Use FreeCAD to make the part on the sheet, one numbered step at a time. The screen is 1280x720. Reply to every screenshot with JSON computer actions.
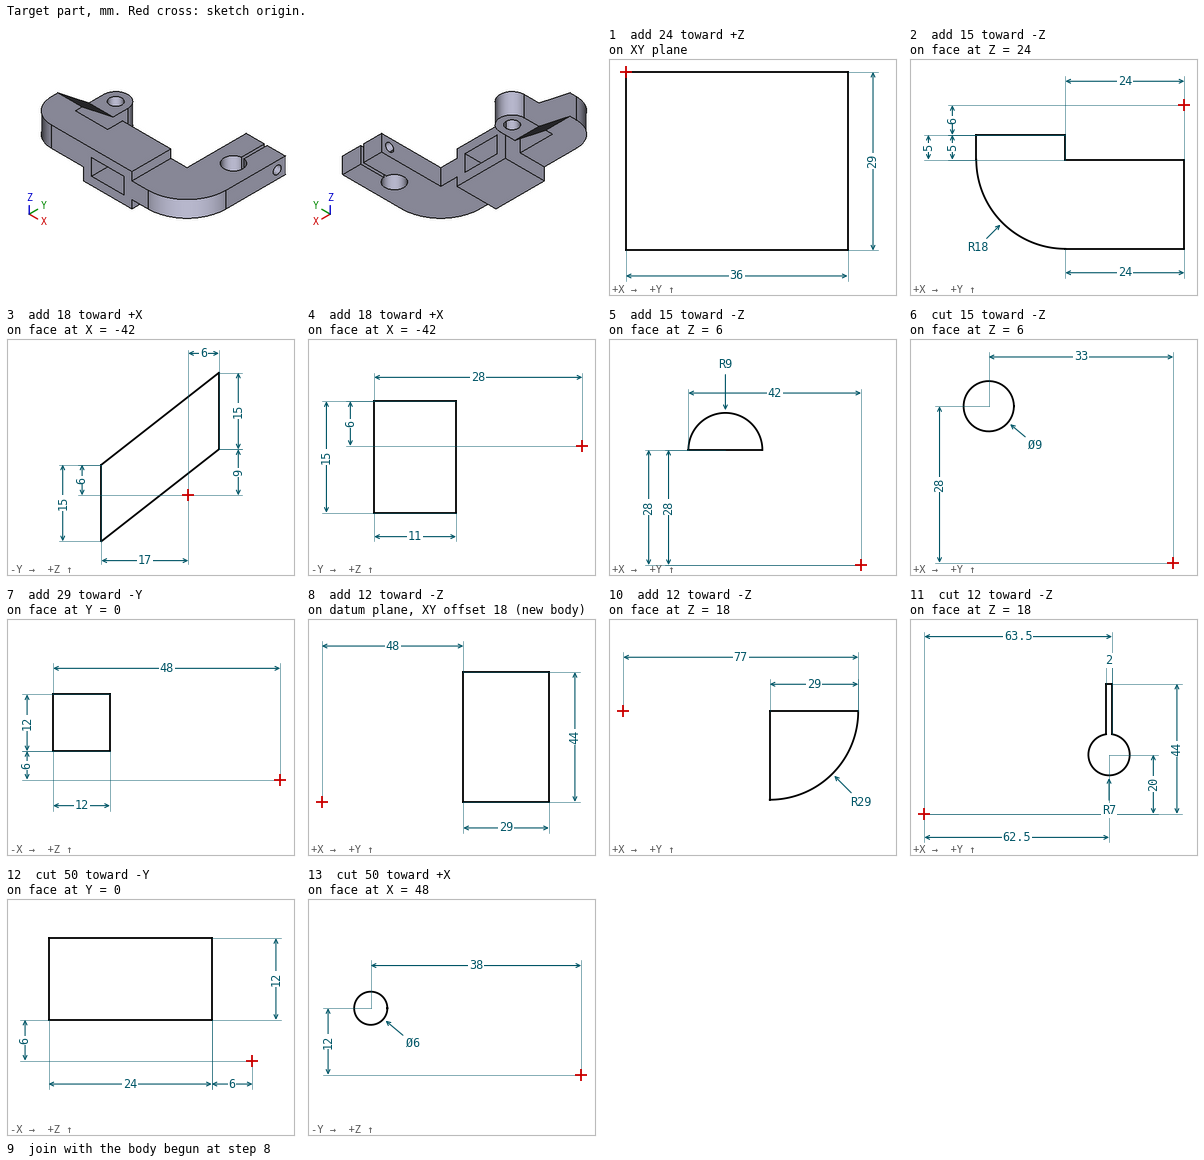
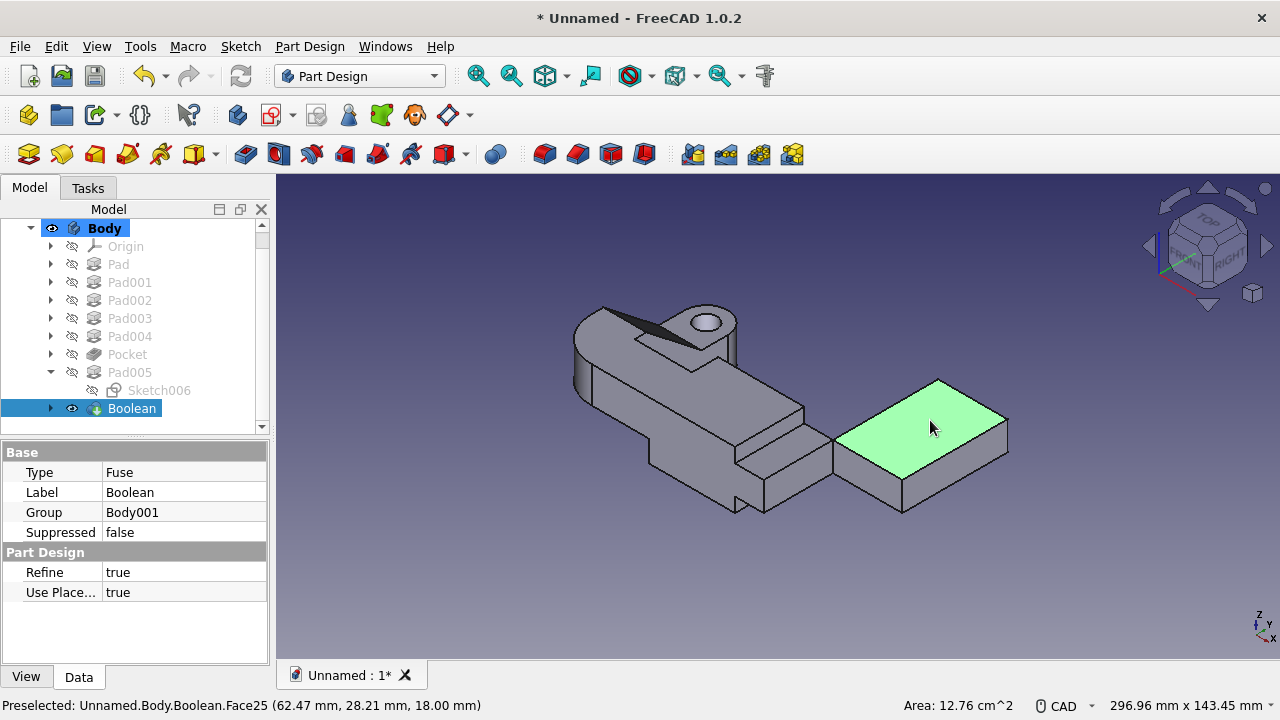
{"action": "left_click", "coordinate": [270, 116]}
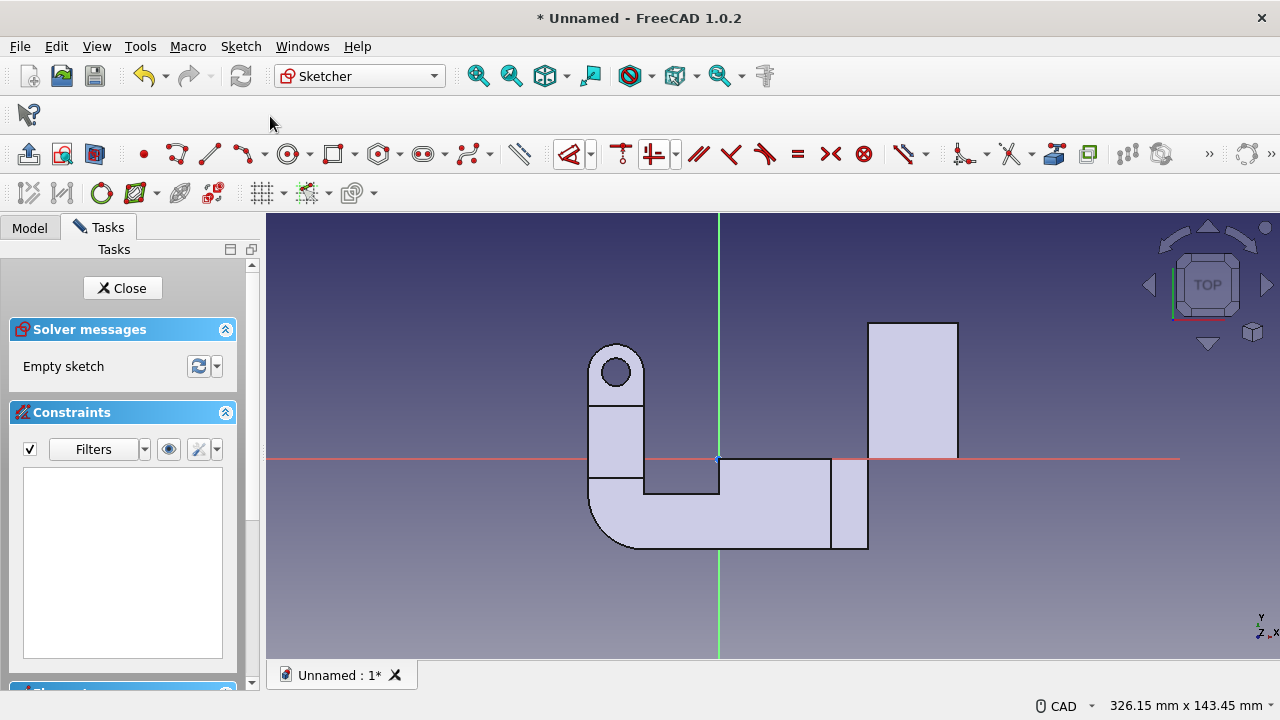
{"action": "scroll", "coordinate": [1003, 534], "scroll_direction": "up", "scroll_amount": 6}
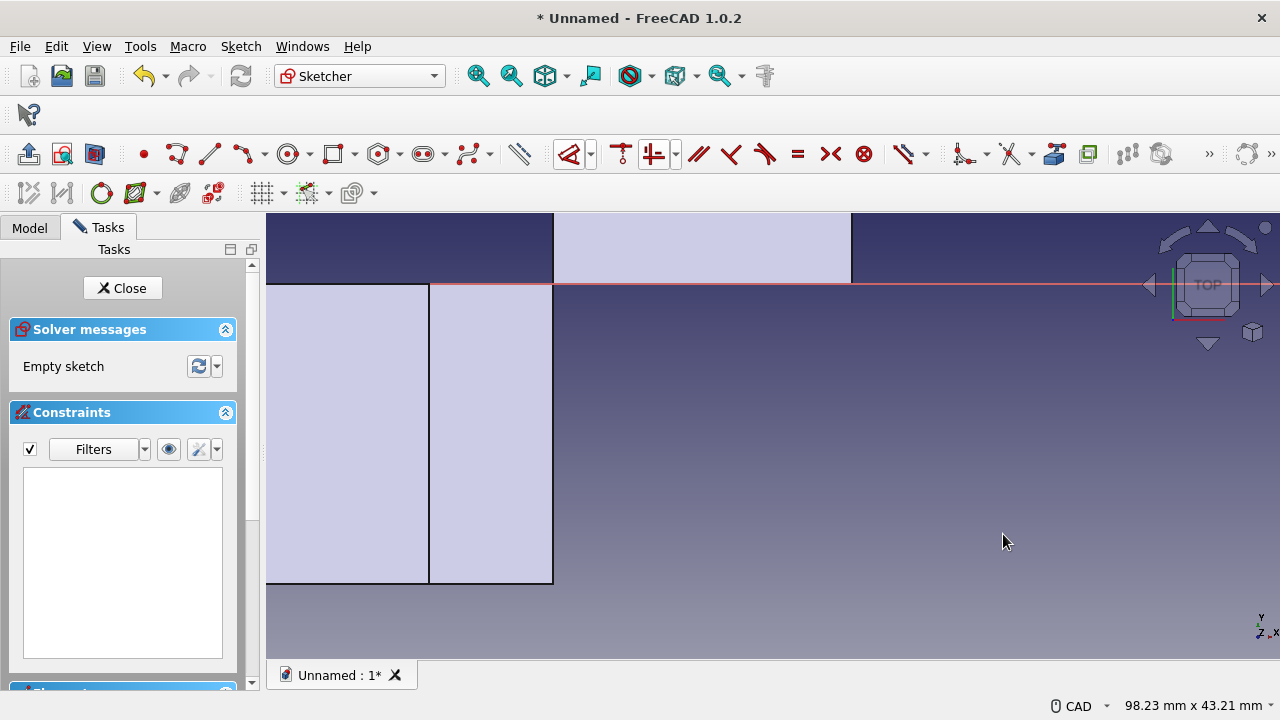
{"action": "left_click", "coordinate": [177, 154]}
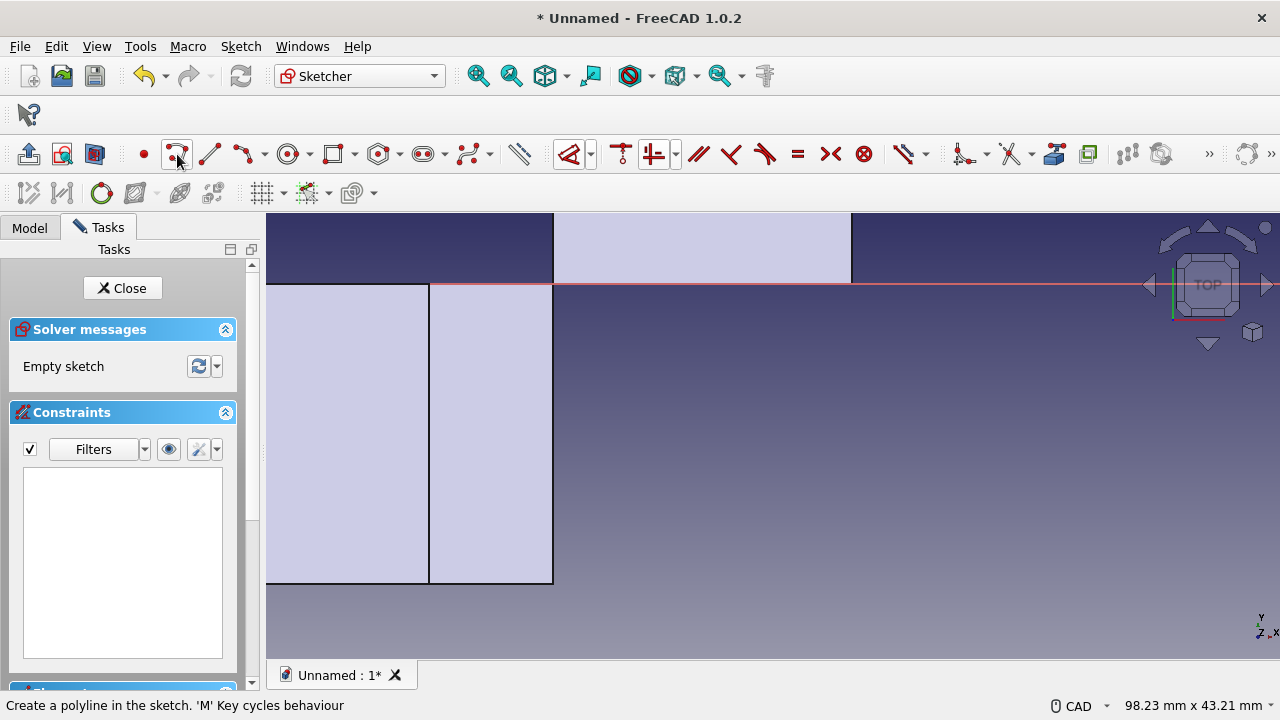
{"action": "left_click", "coordinate": [852, 284]}
{"action": "left_click", "coordinate": [553, 293]}
{"action": "left_click", "coordinate": [553, 584]}
{"action": "right_click", "coordinate": [553, 584]}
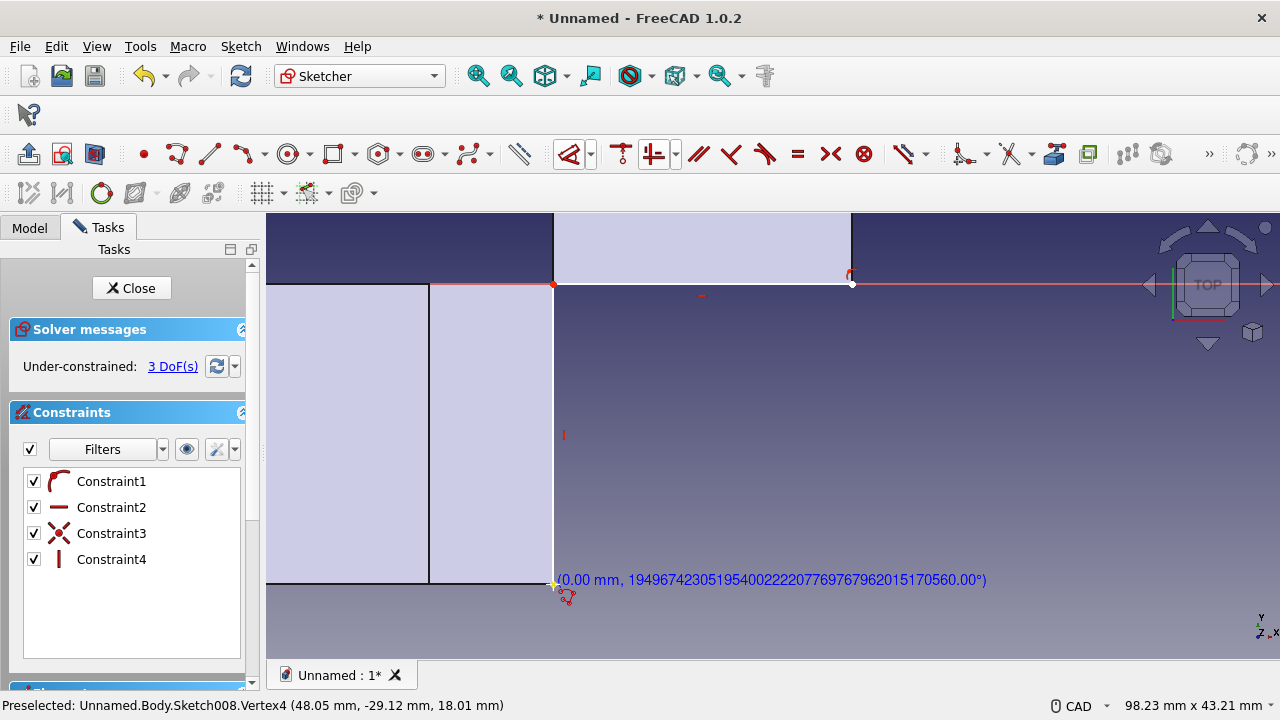
{"action": "left_click", "coordinate": [242, 154]}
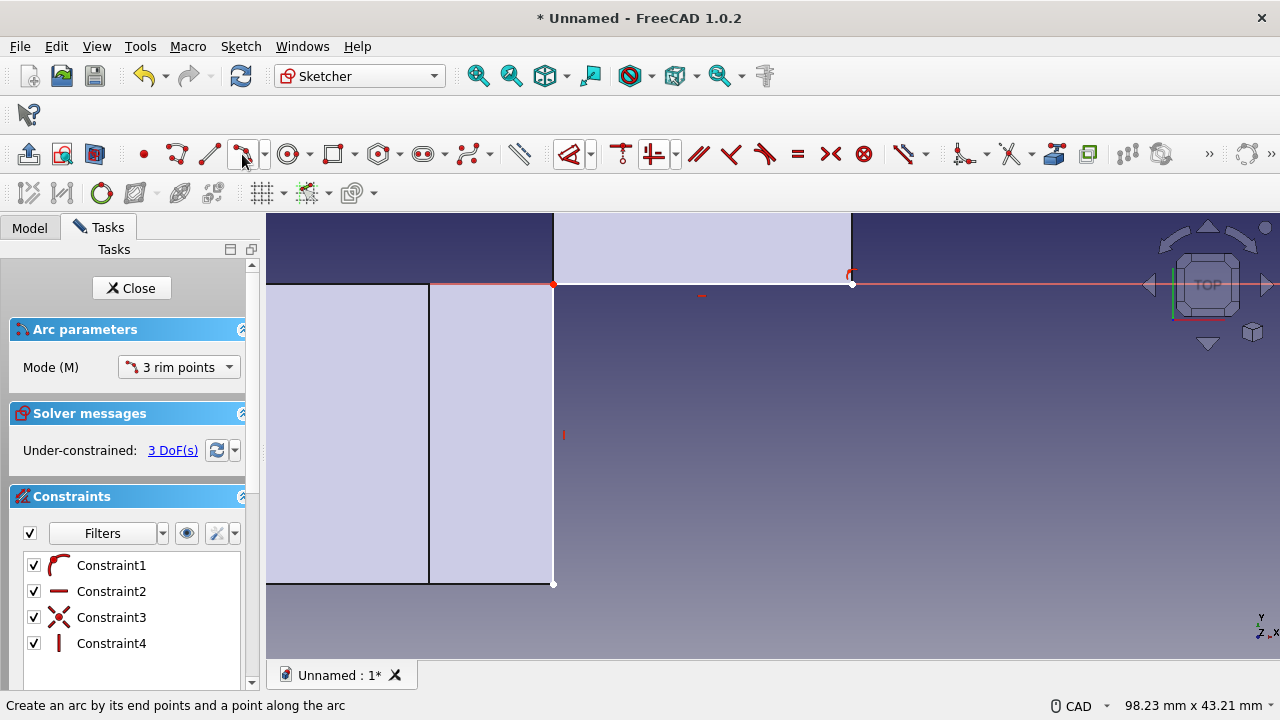
{"action": "left_click", "coordinate": [553, 585]}
{"action": "left_click", "coordinate": [852, 284]}
{"action": "left_click", "coordinate": [764, 496]}
{"action": "key", "text": "Escape"}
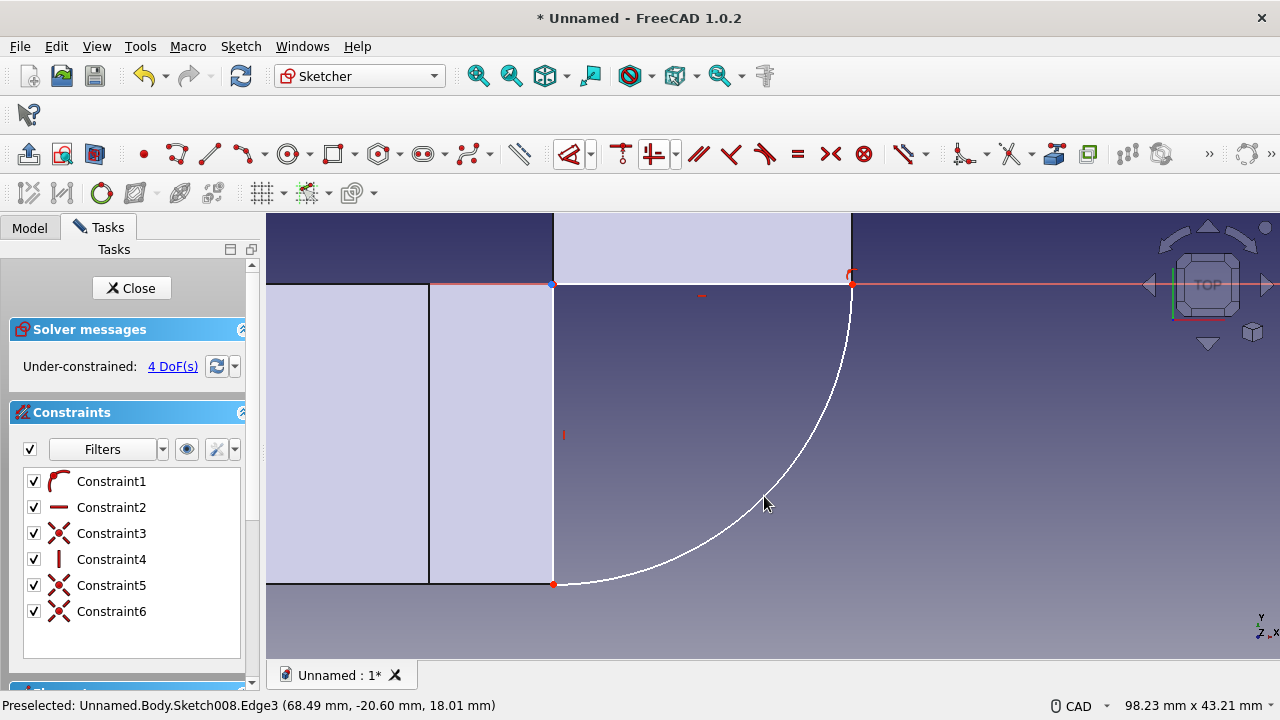
{"action": "left_click", "coordinate": [552, 285]}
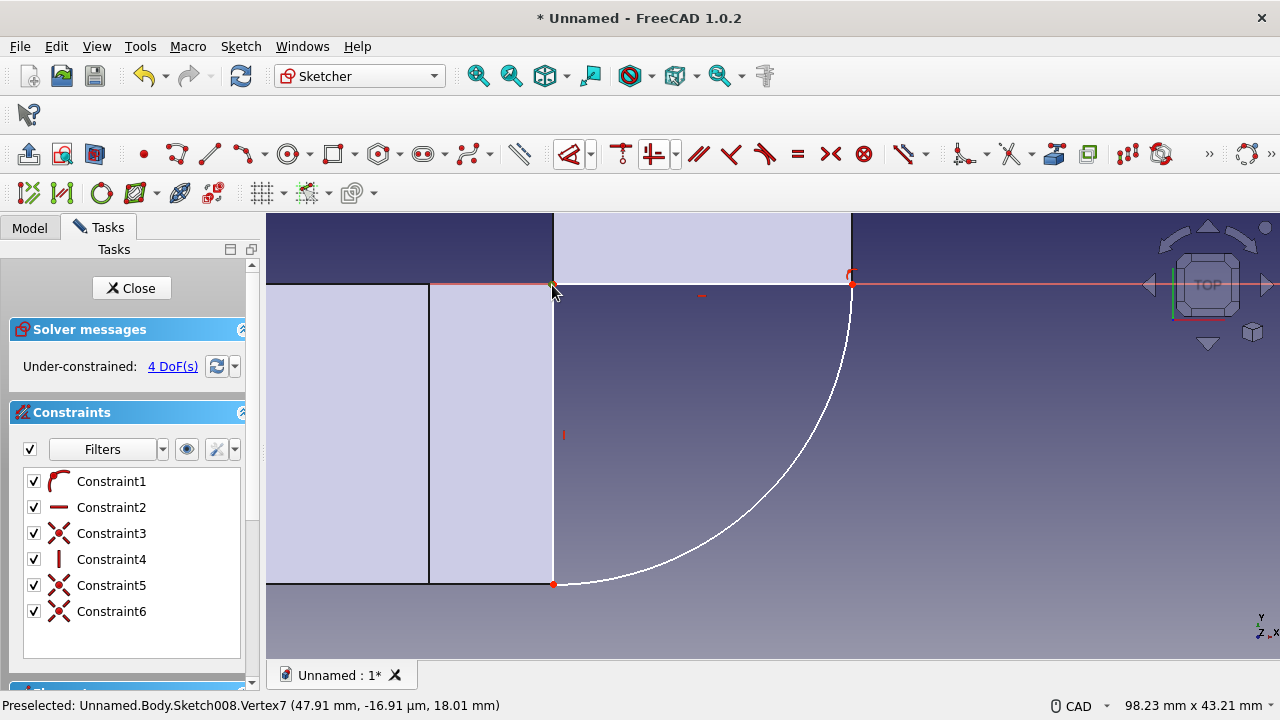
{"action": "left_click", "coordinate": [353, 284]}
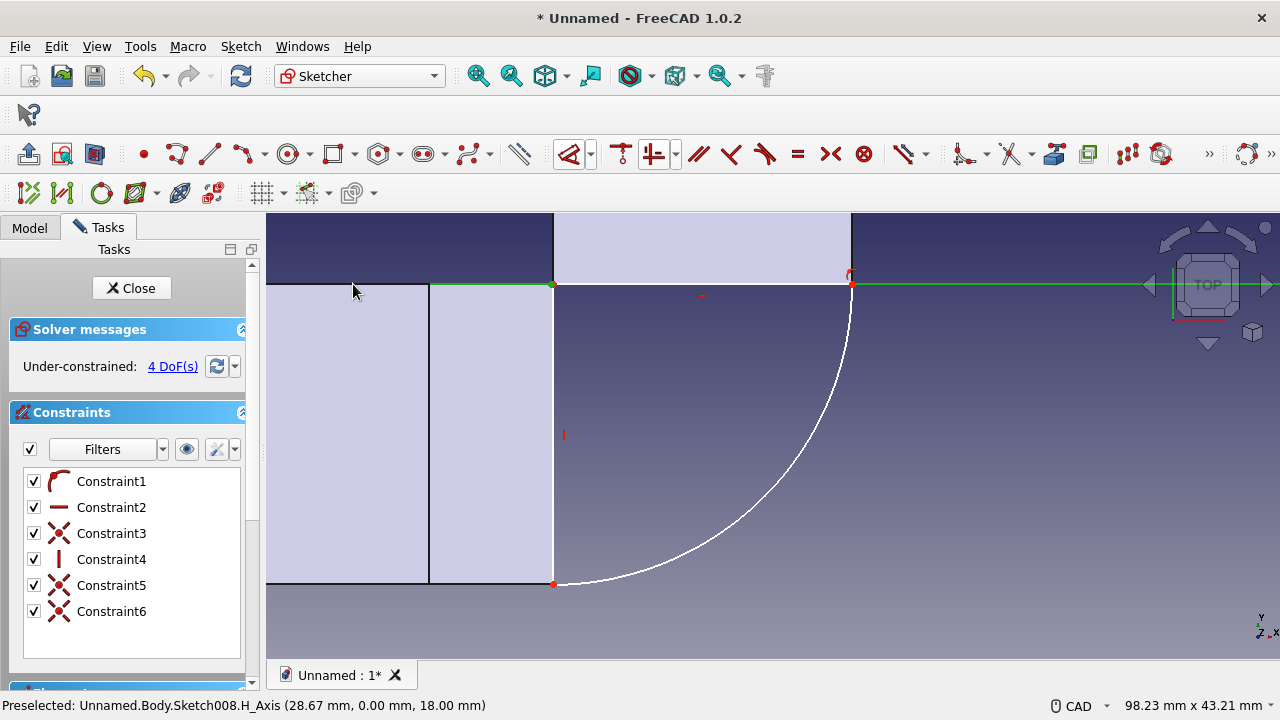
{"action": "left_click", "coordinate": [621, 154]}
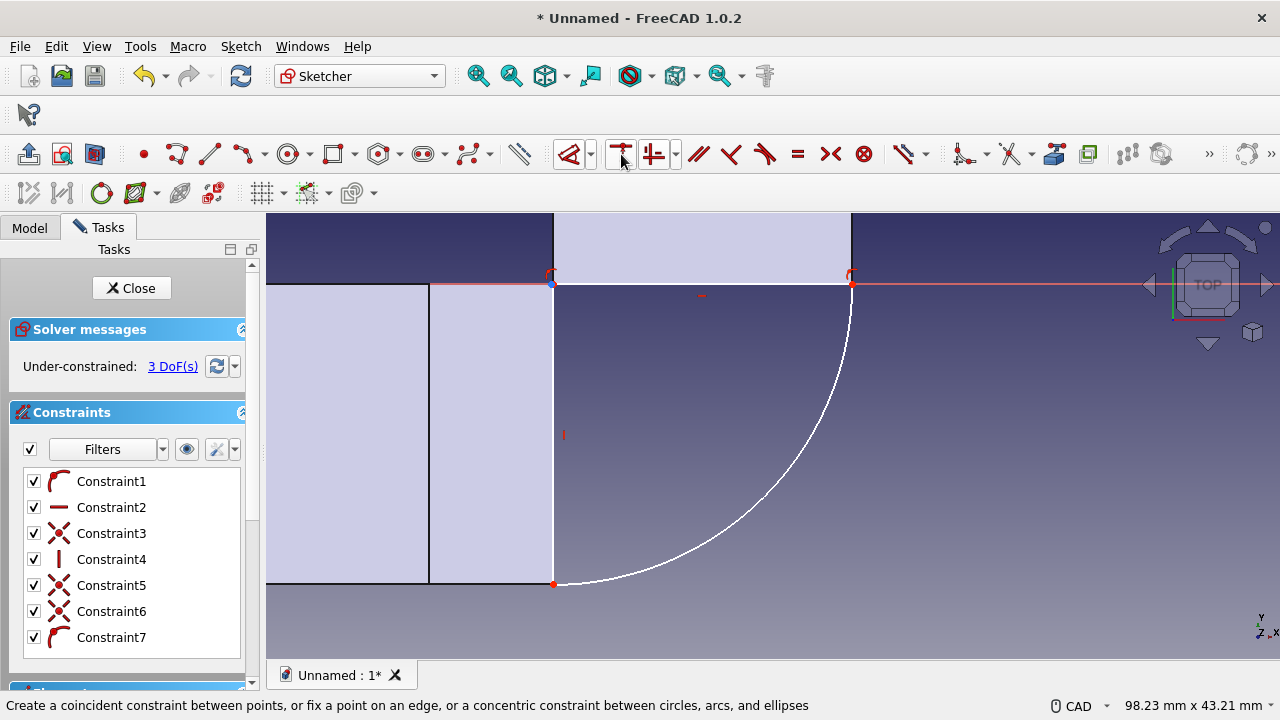
{"action": "left_click", "coordinate": [689, 552]}